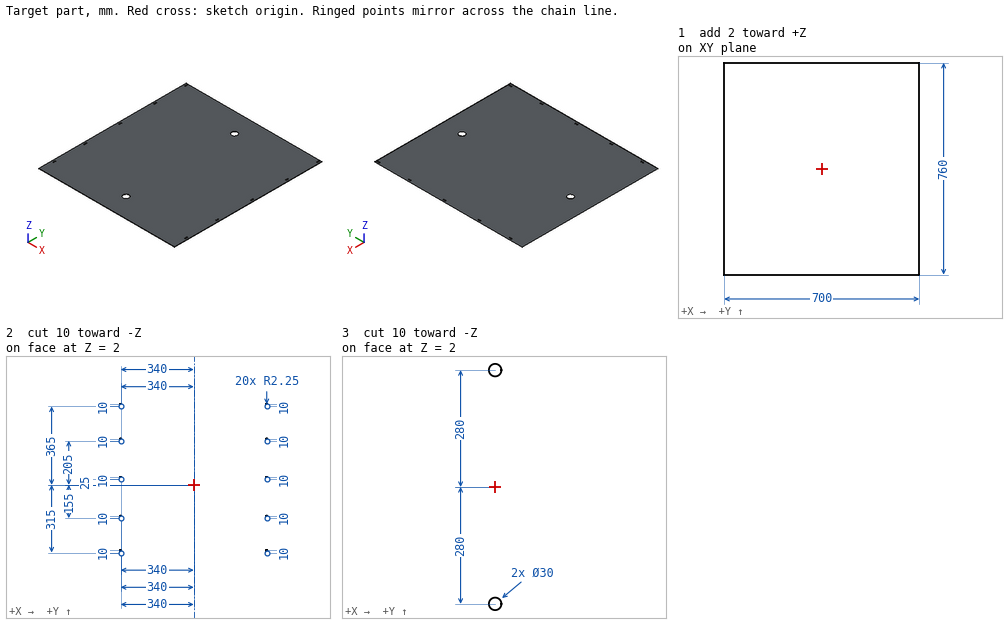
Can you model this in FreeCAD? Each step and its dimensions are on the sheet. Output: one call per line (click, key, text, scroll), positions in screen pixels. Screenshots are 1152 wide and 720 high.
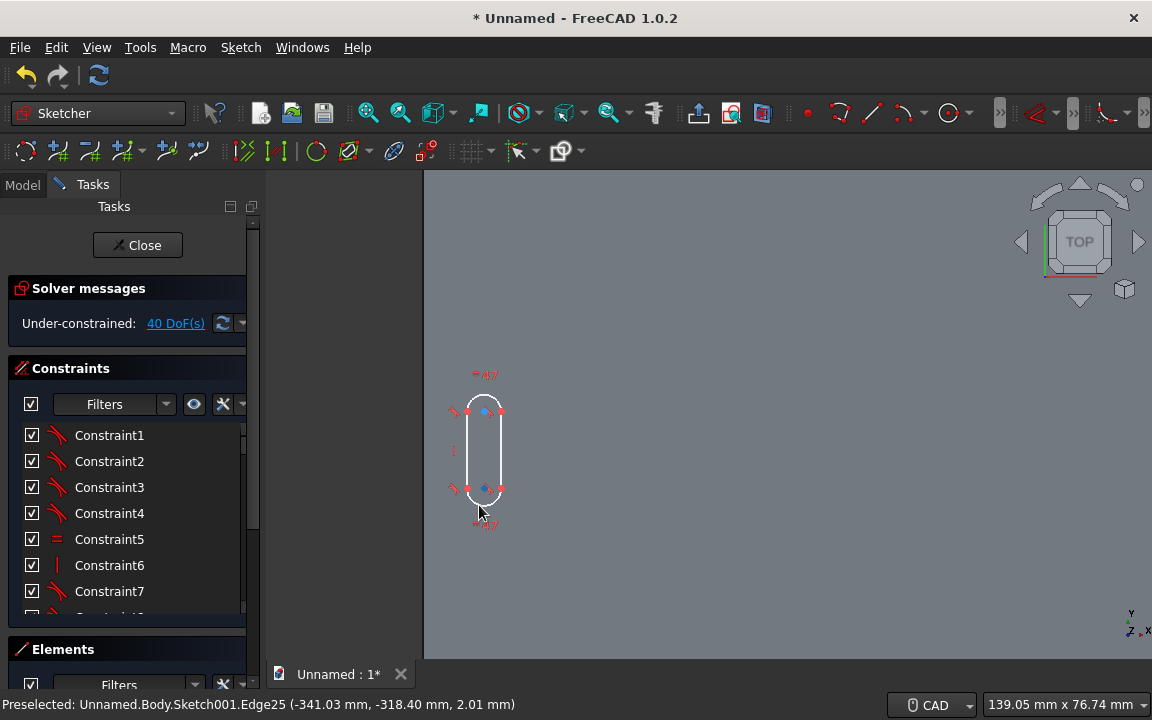
click(474, 503)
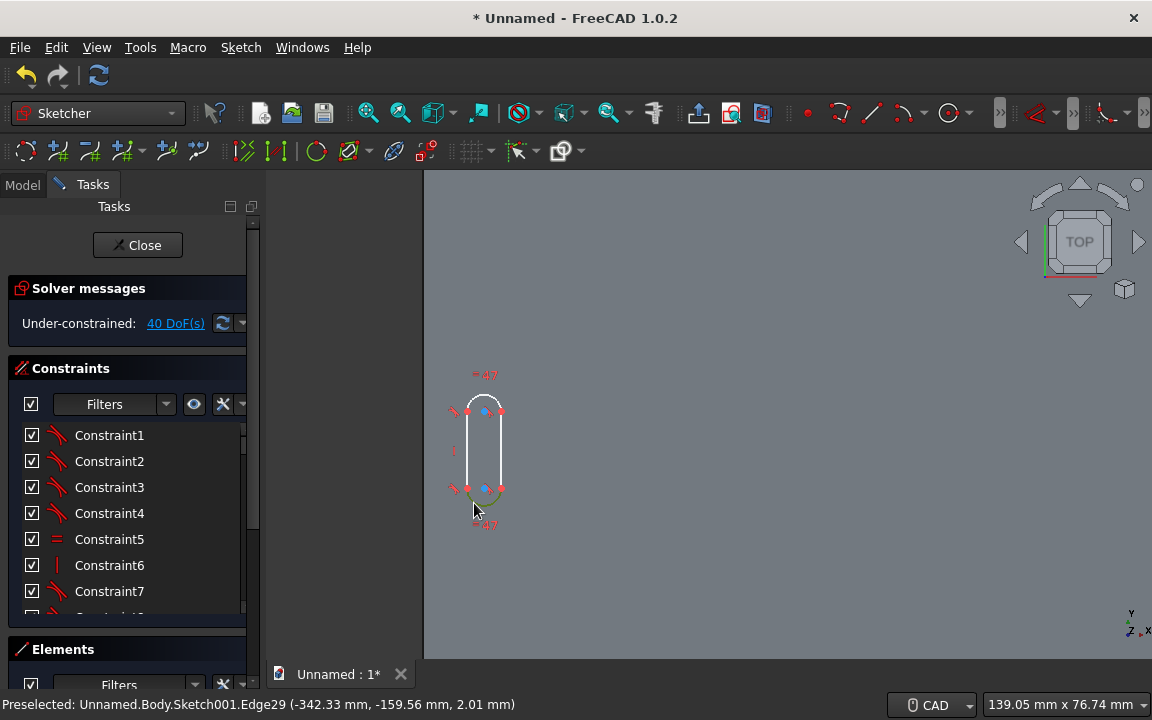
scroll(479, 505, down, 13)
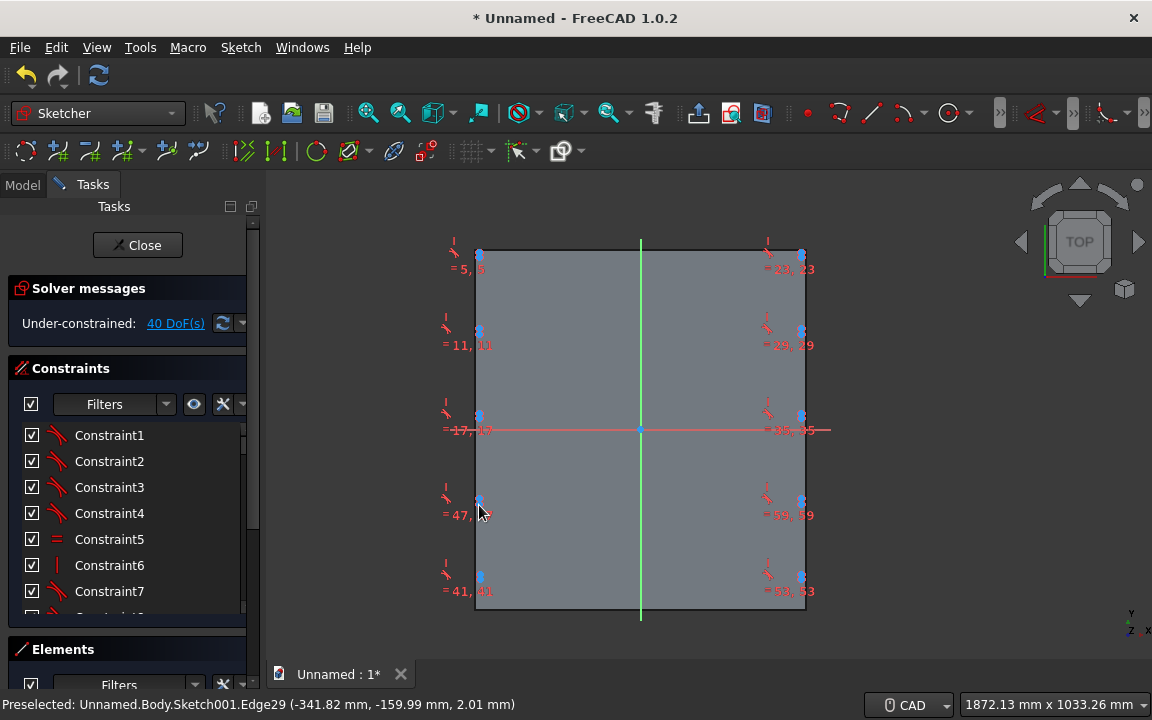
scroll(801, 581, up, 14)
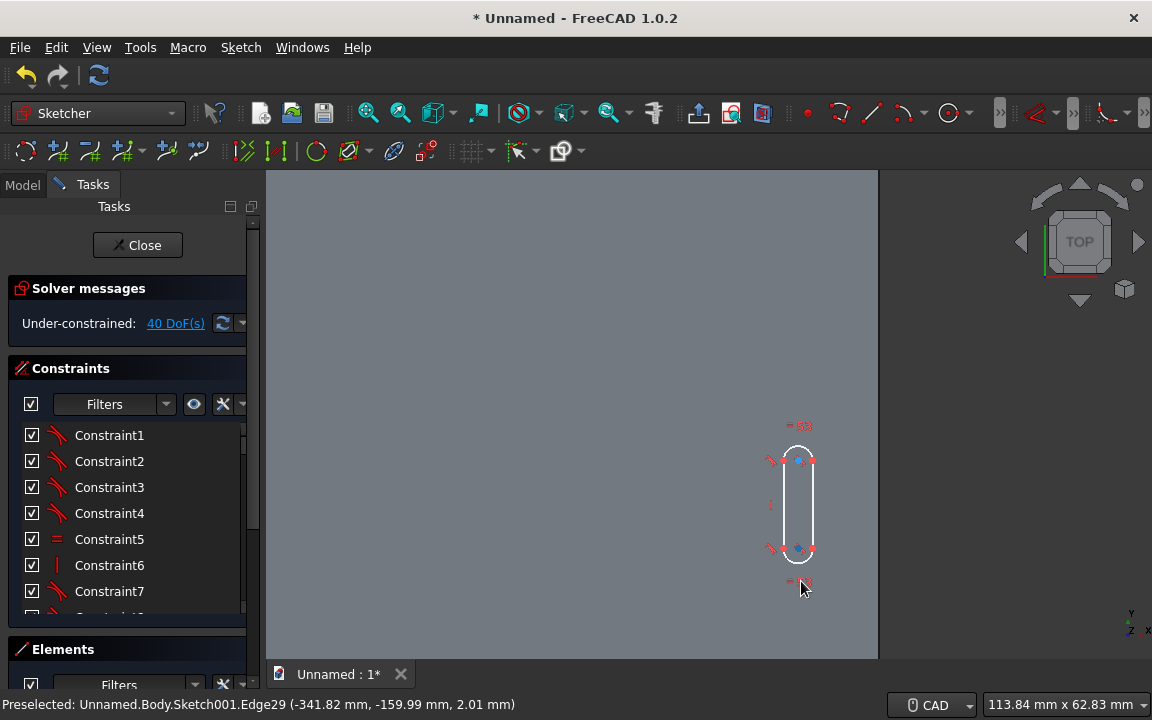
click(790, 561)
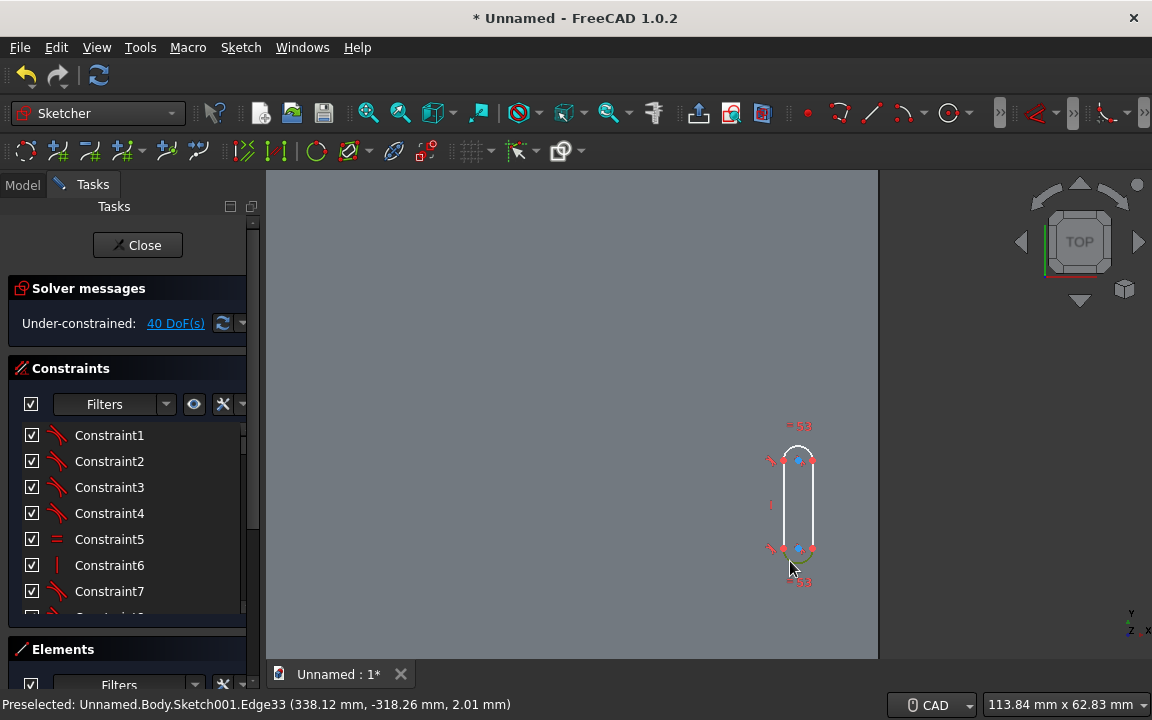
scroll(801, 581, down, 14)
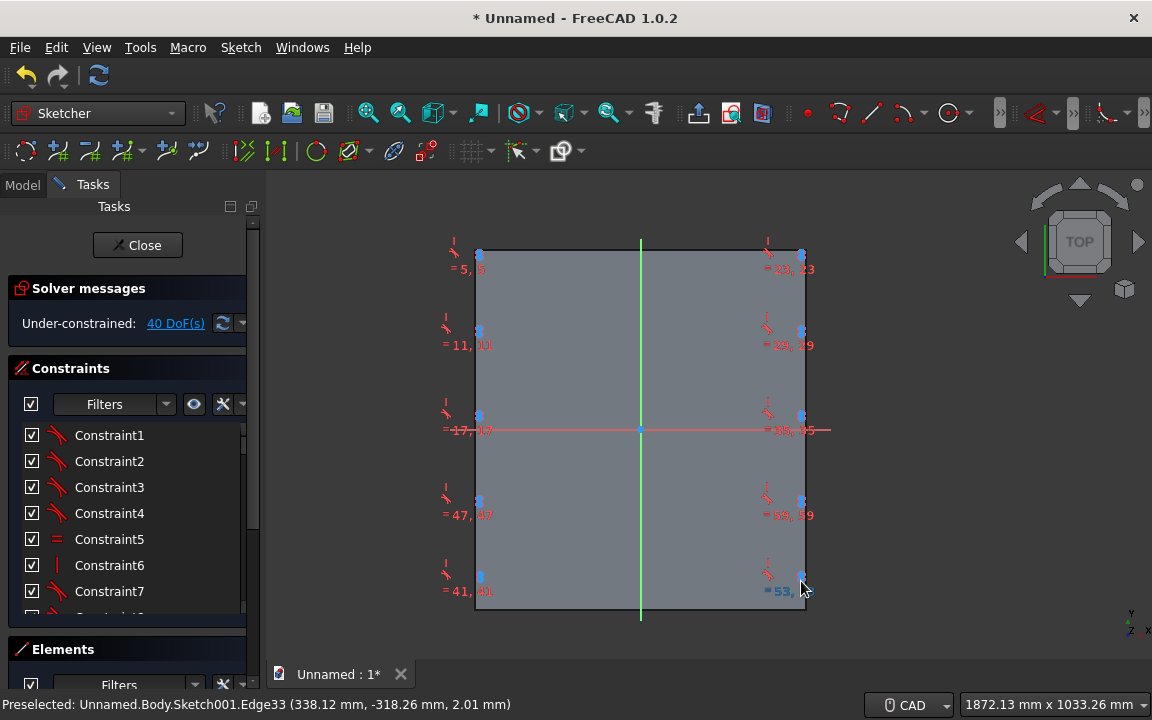
scroll(801, 505, up, 13)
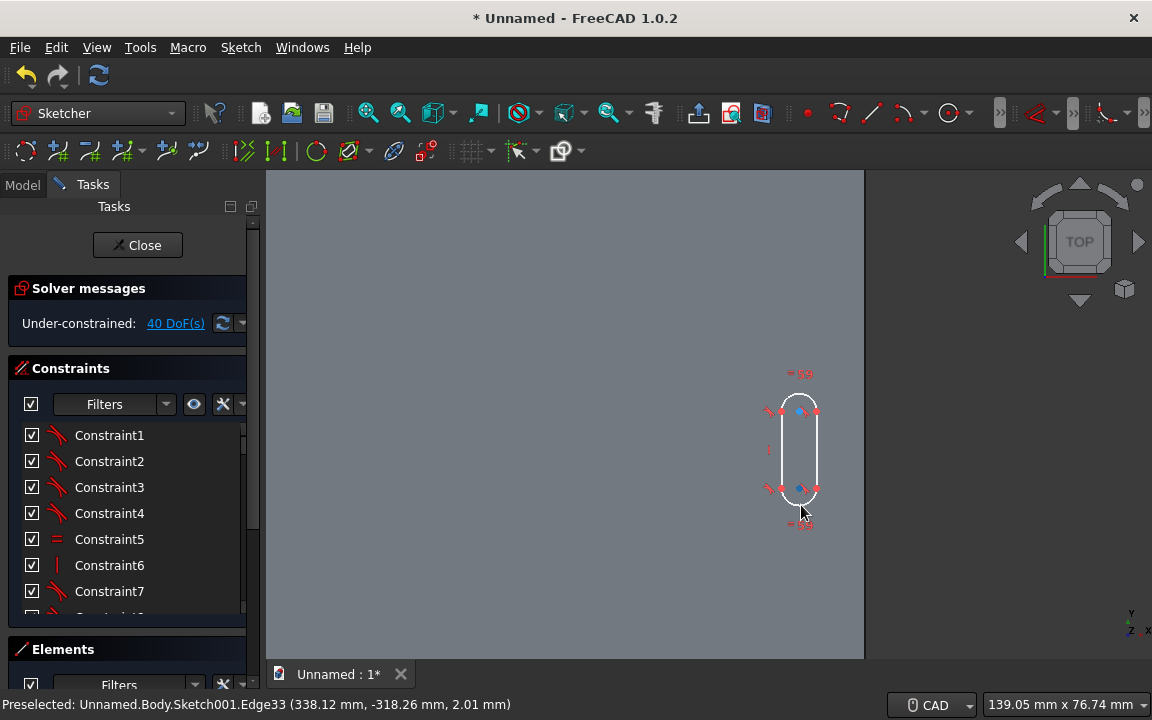
click(789, 502)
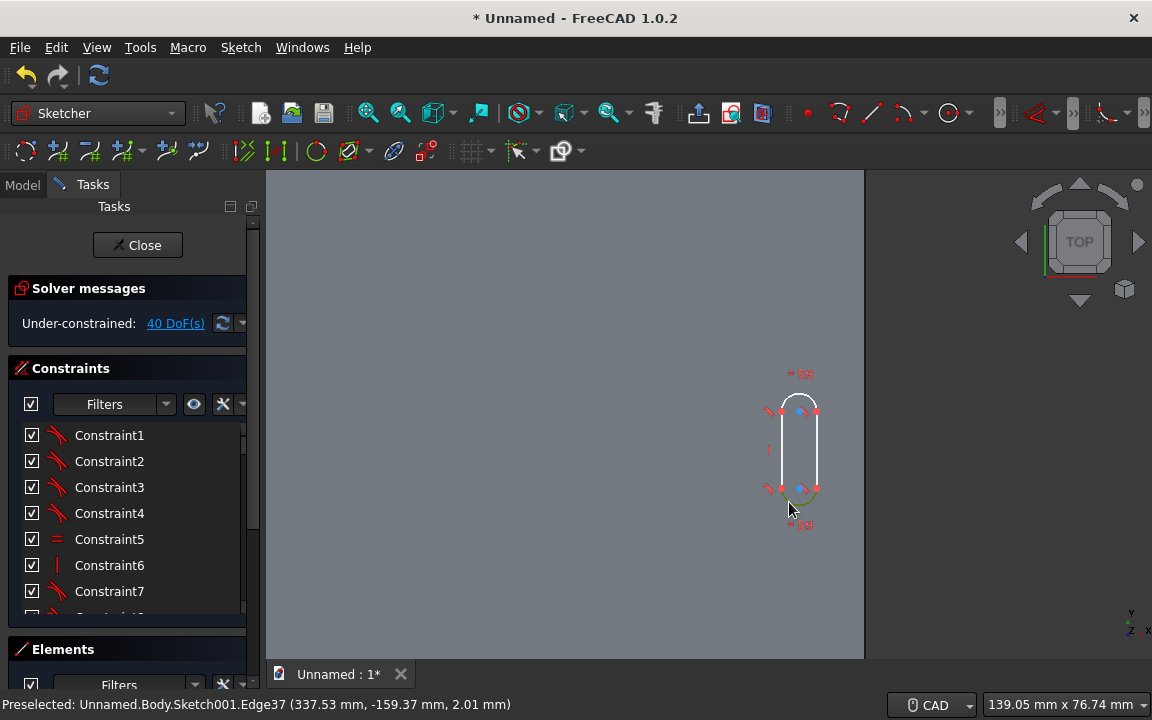
key(e)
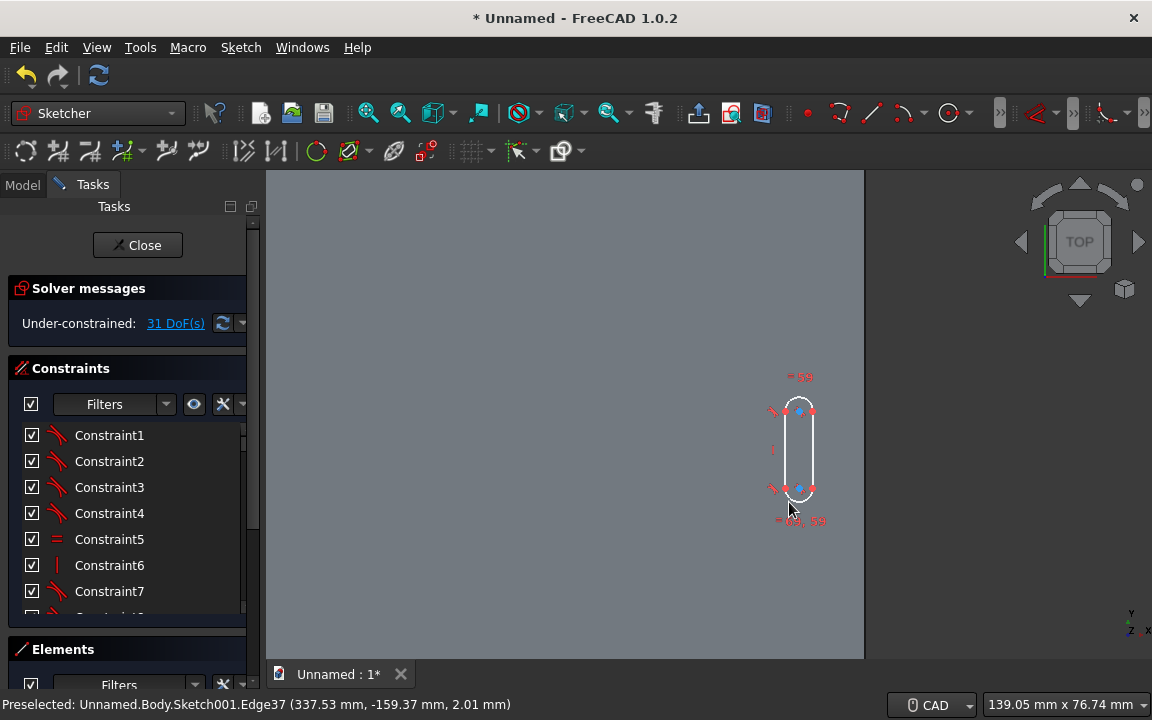
scroll(801, 505, down, 13)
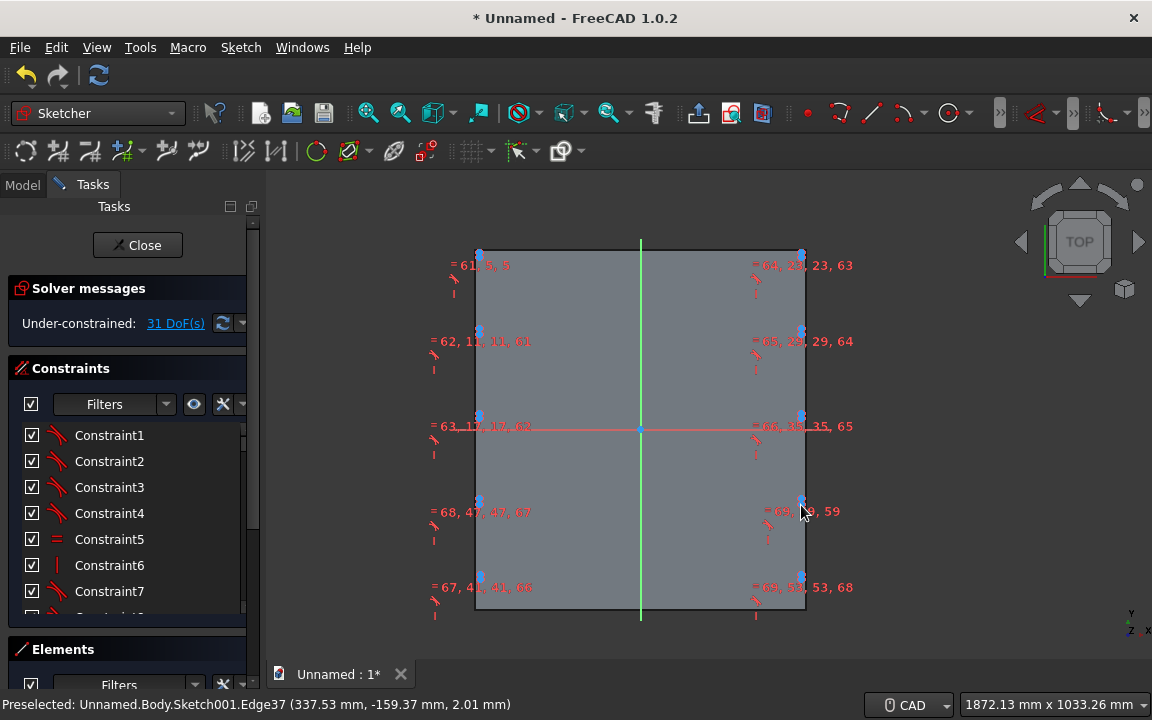
scroll(480, 258, up, 13)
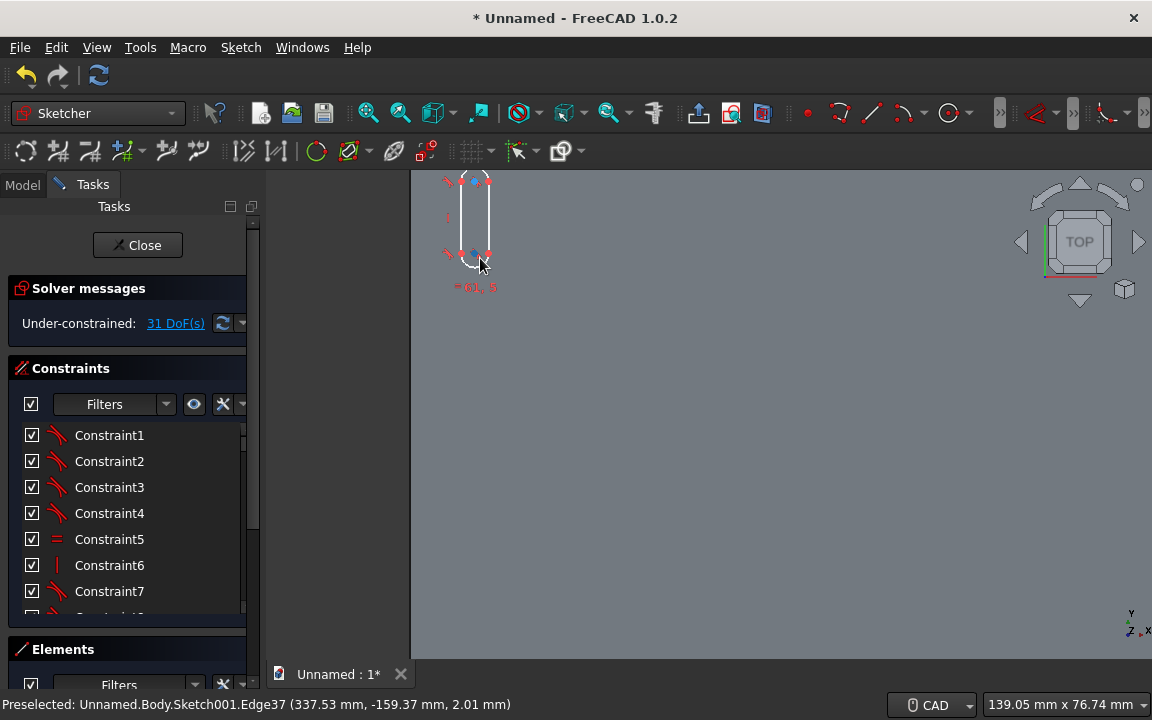
click(475, 254)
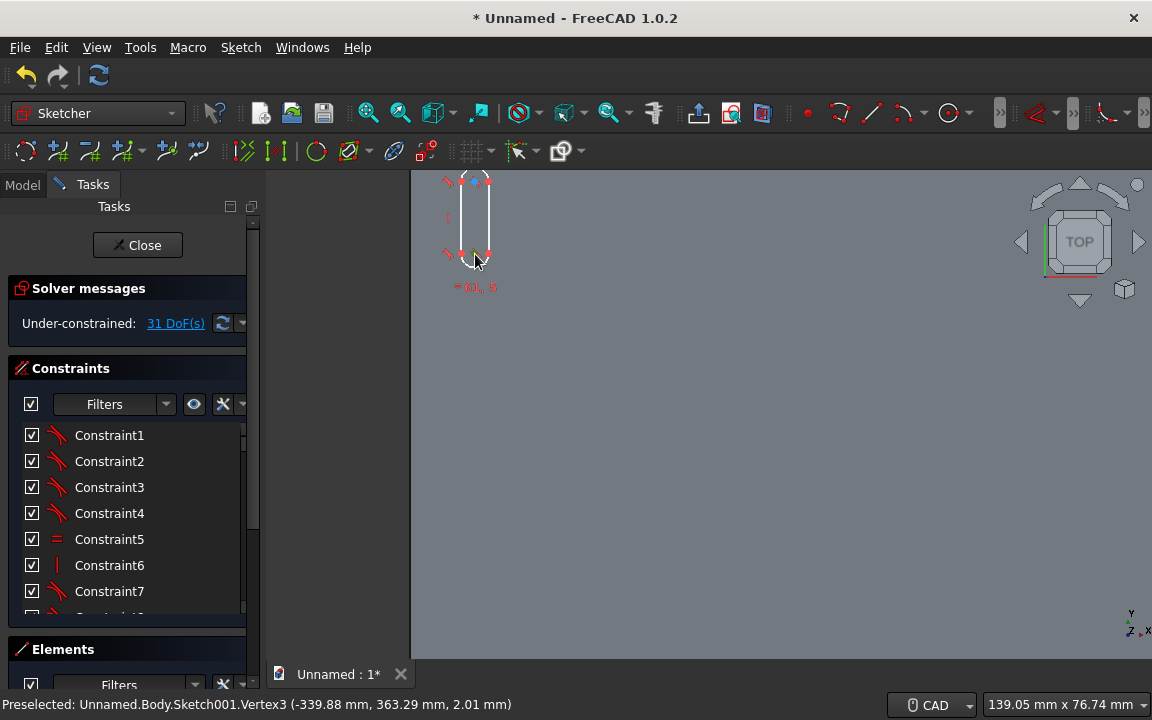
scroll(480, 257, down, 13)